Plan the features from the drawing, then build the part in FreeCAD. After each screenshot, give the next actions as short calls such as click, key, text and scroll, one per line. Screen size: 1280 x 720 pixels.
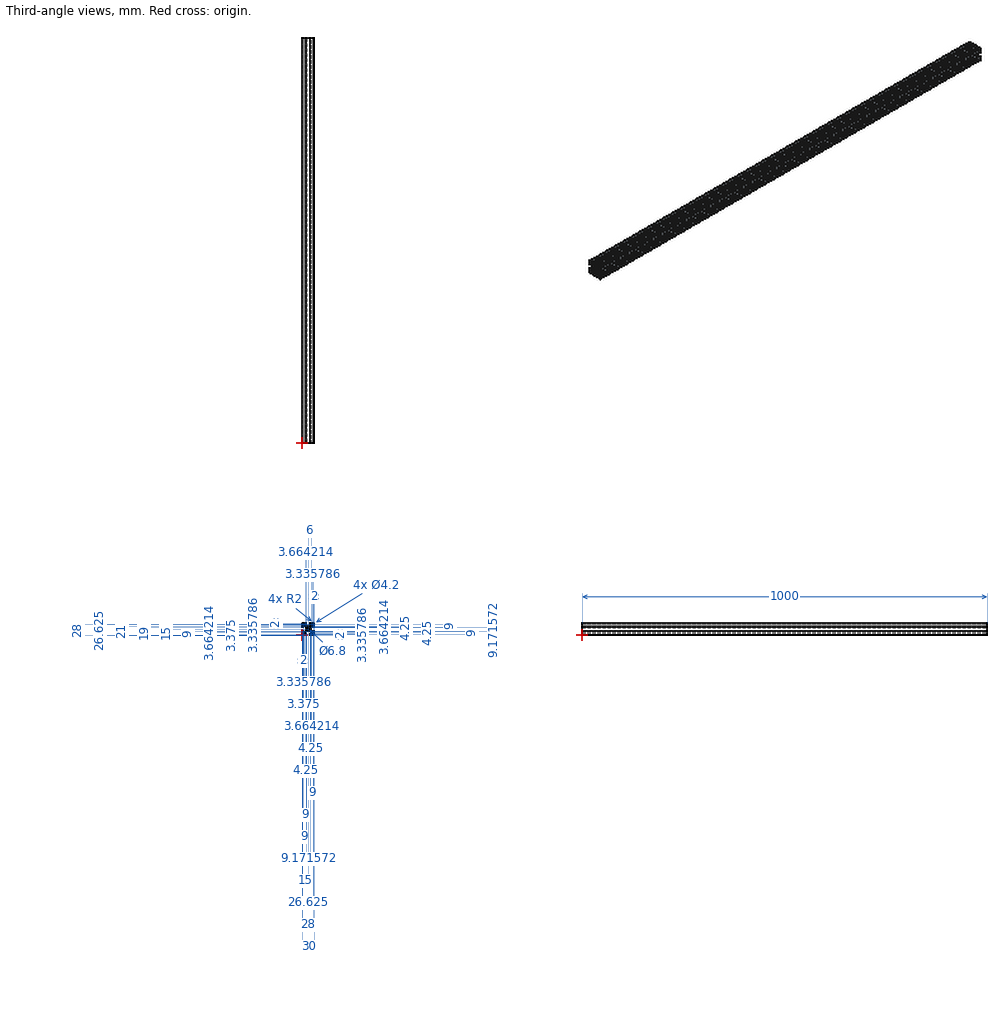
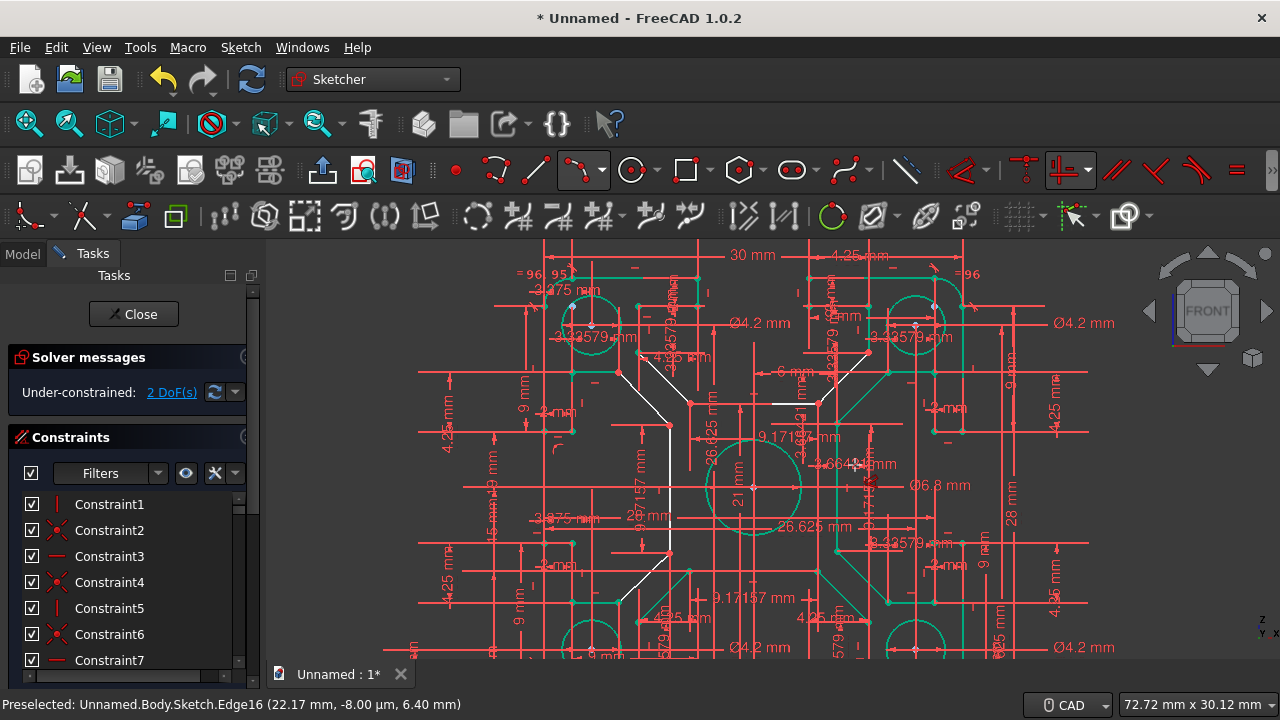
click(634, 588)
click(439, 595)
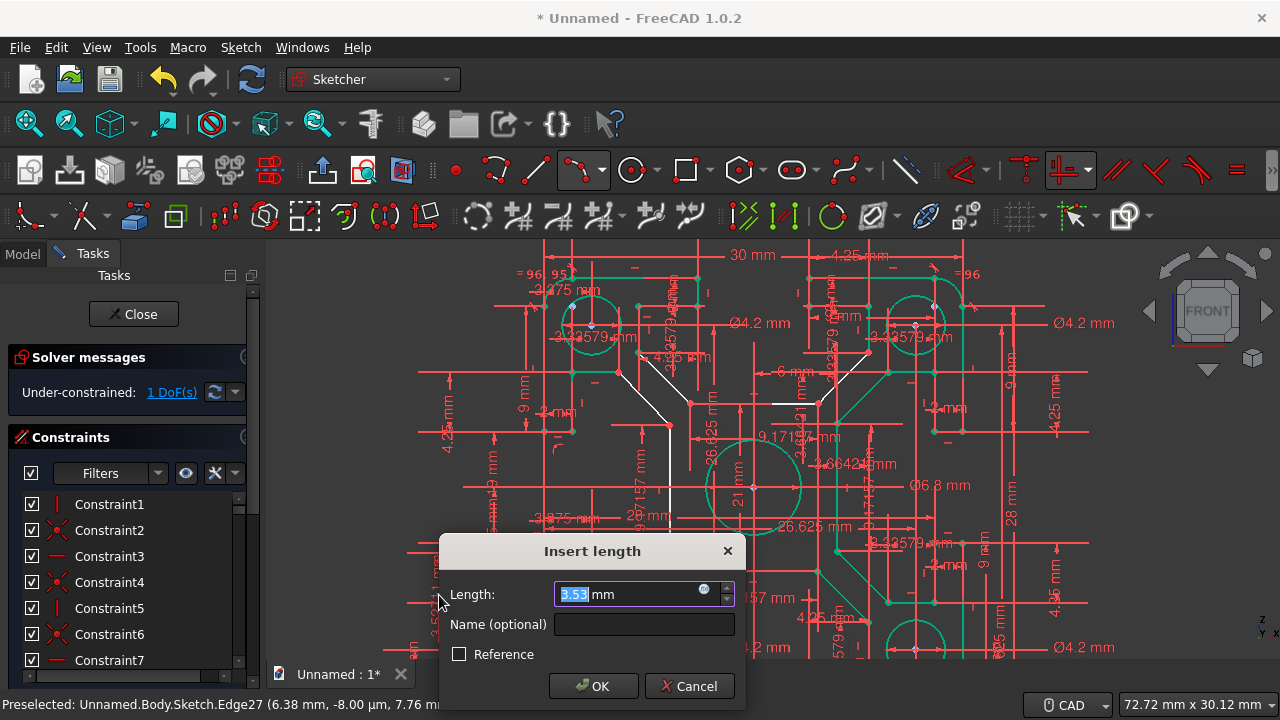
text(3.664214)
key(Return)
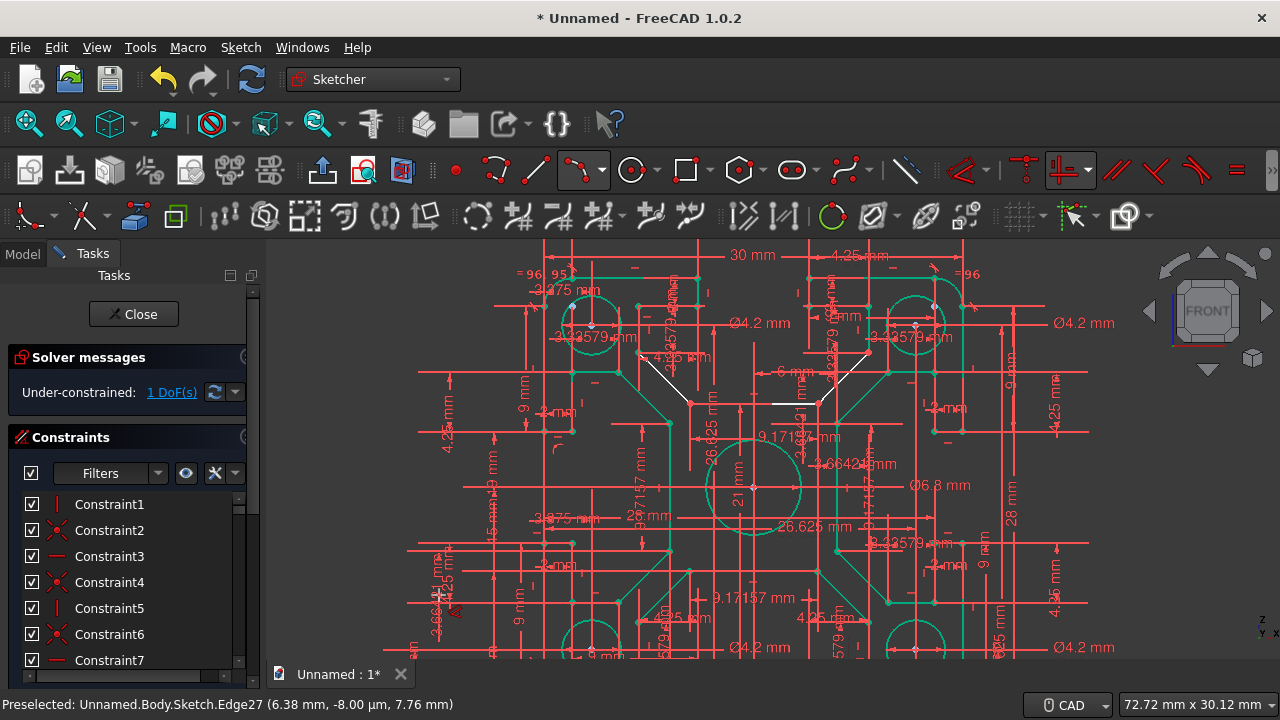
click(654, 368)
click(653, 462)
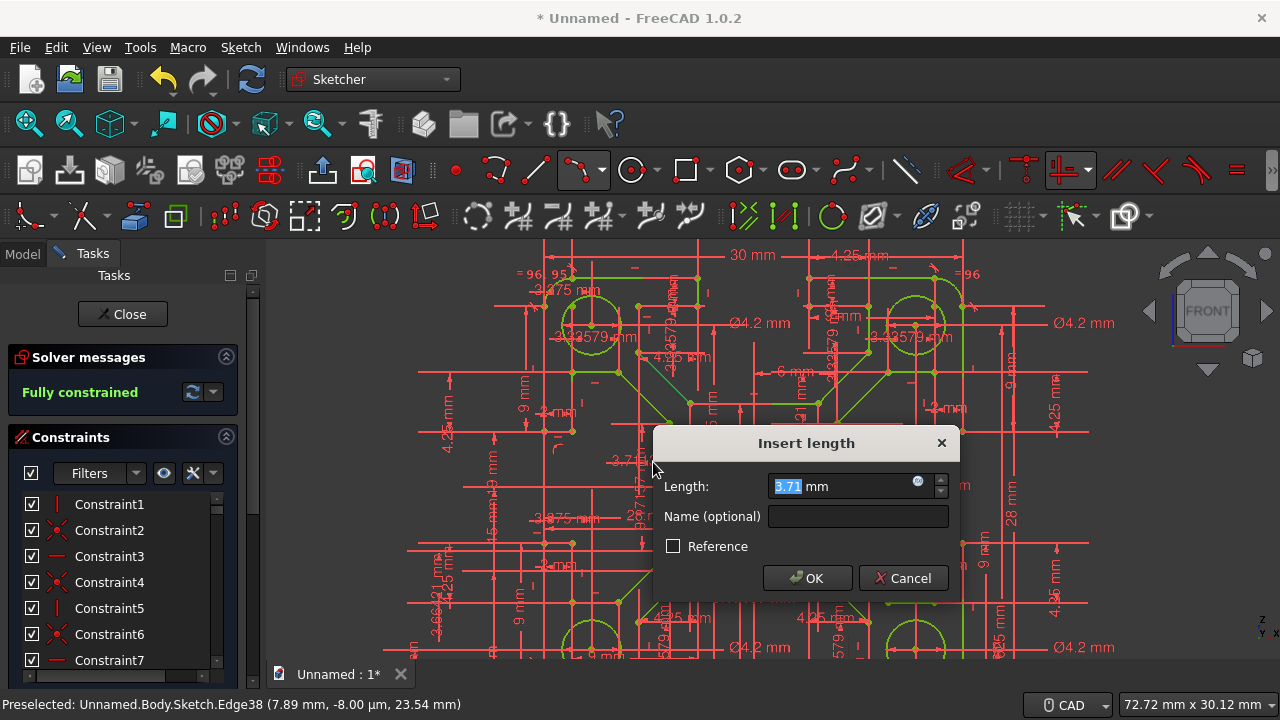
text(3.664214)
key(Return)
key(Escape)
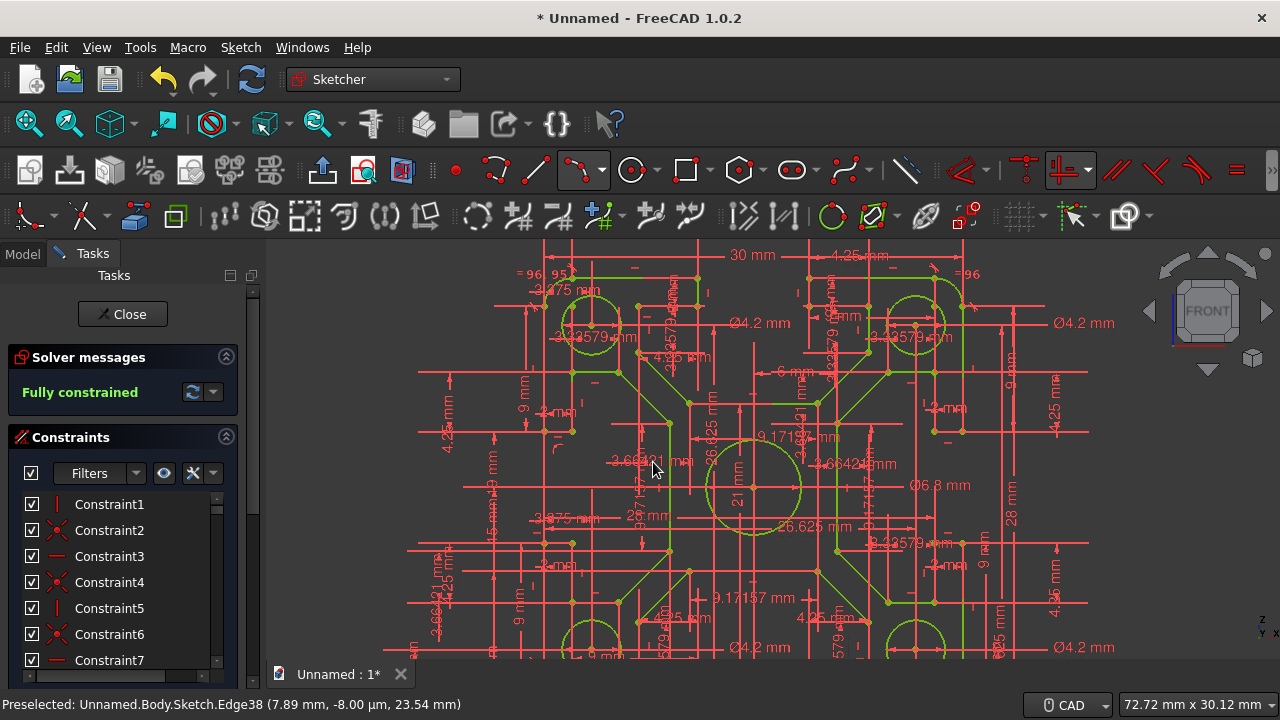
click(123, 314)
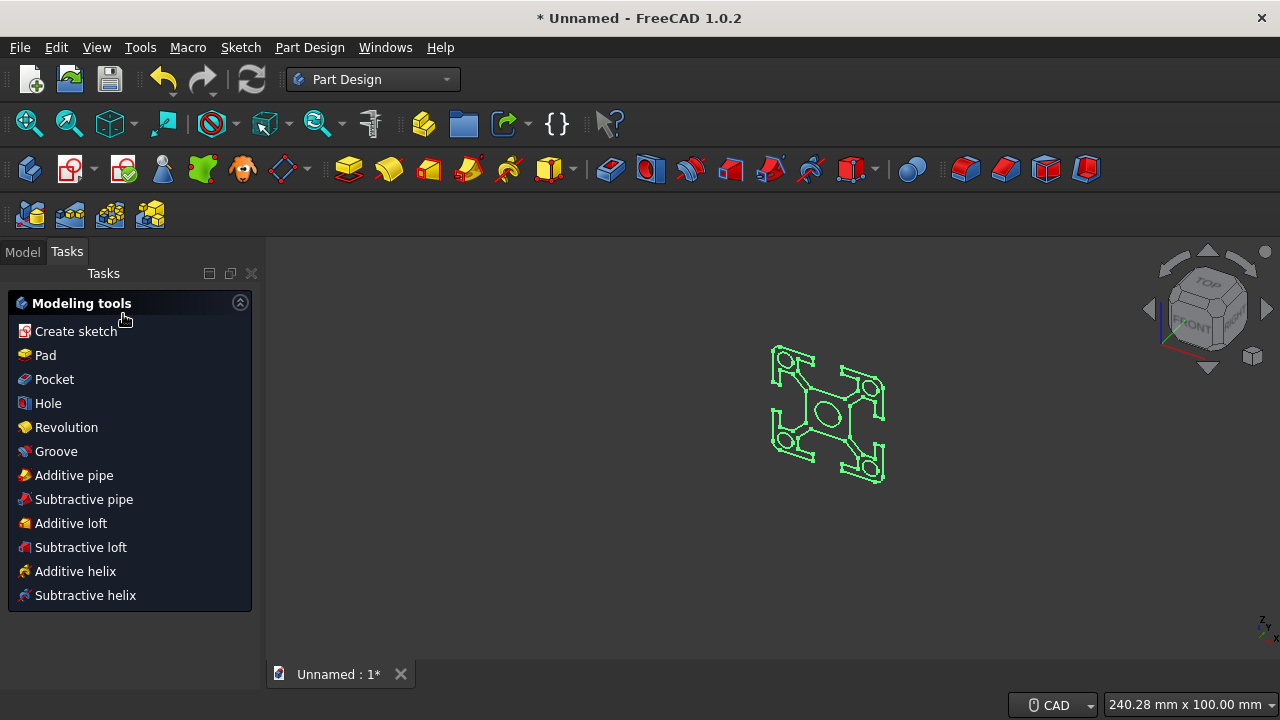
click(350, 170)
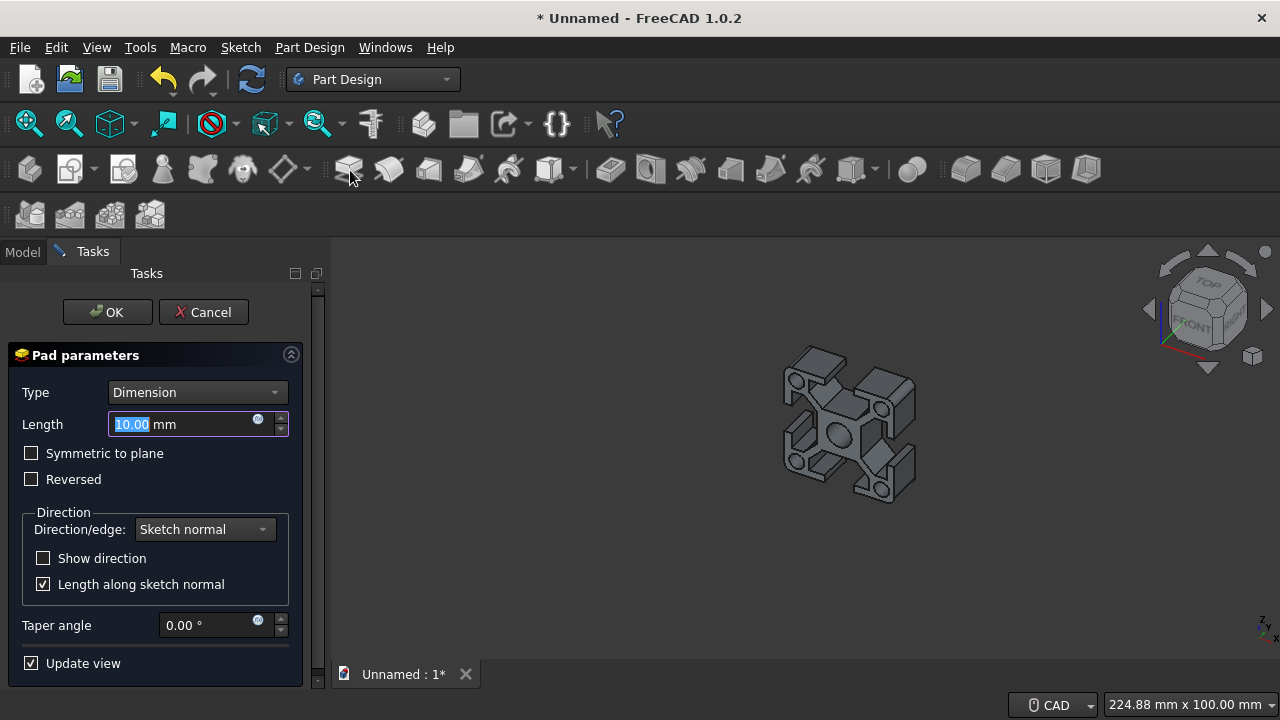
text(1000)
key(Tab)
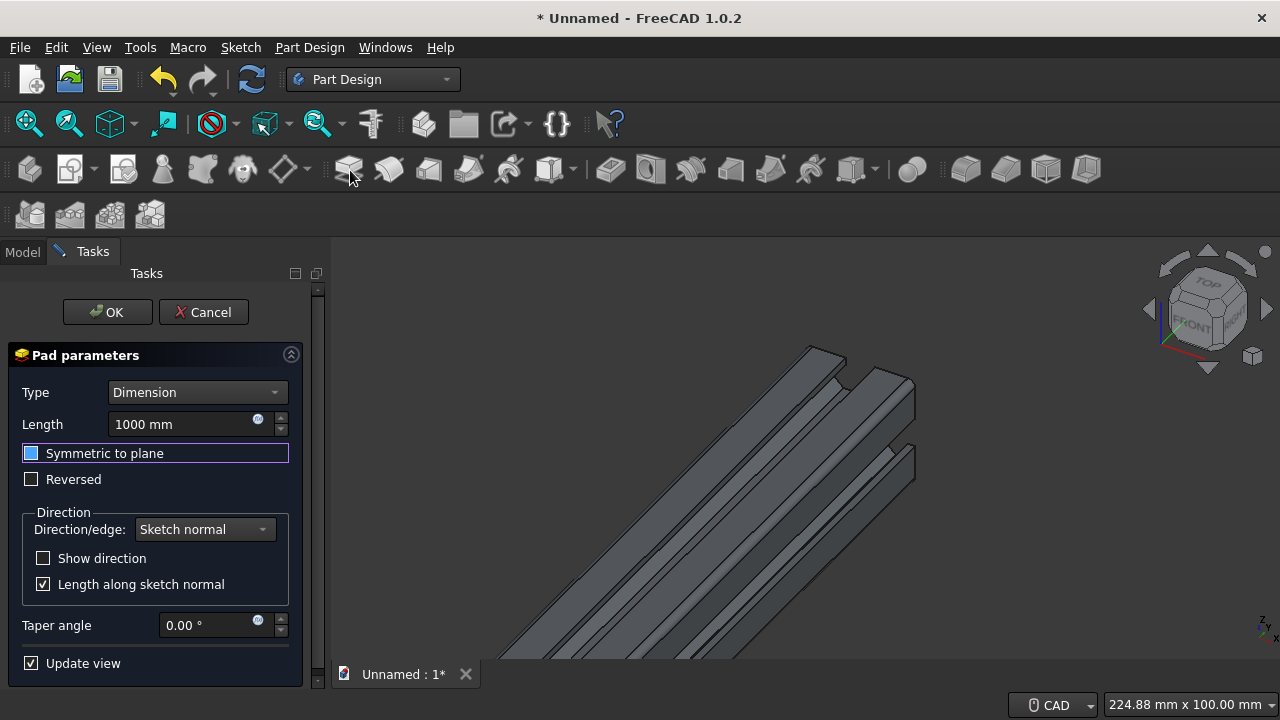
click(30, 479)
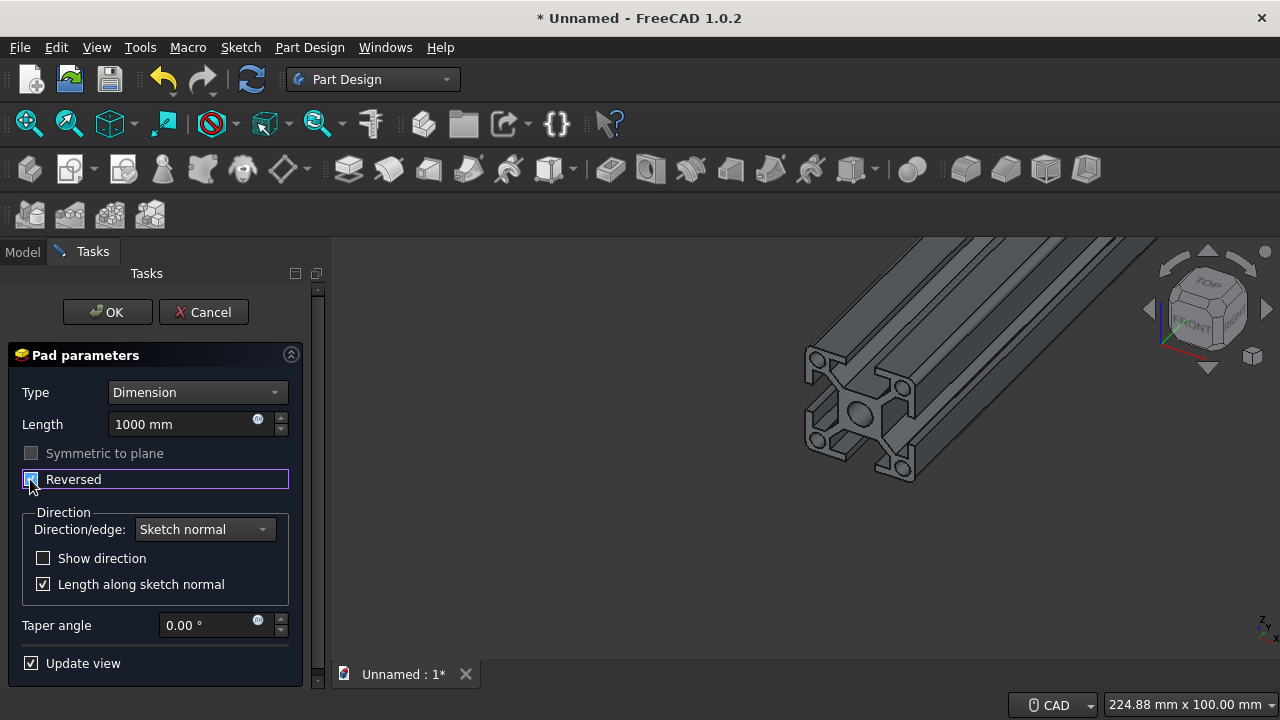
click(108, 312)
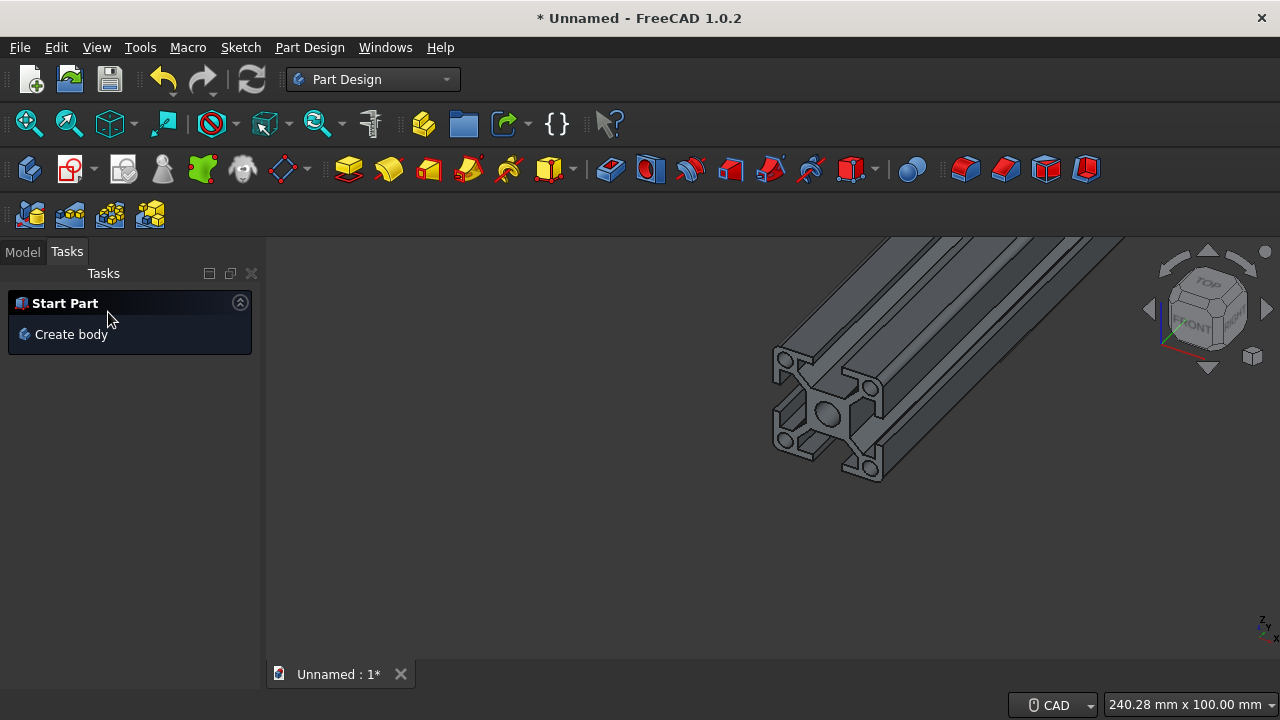
key(0)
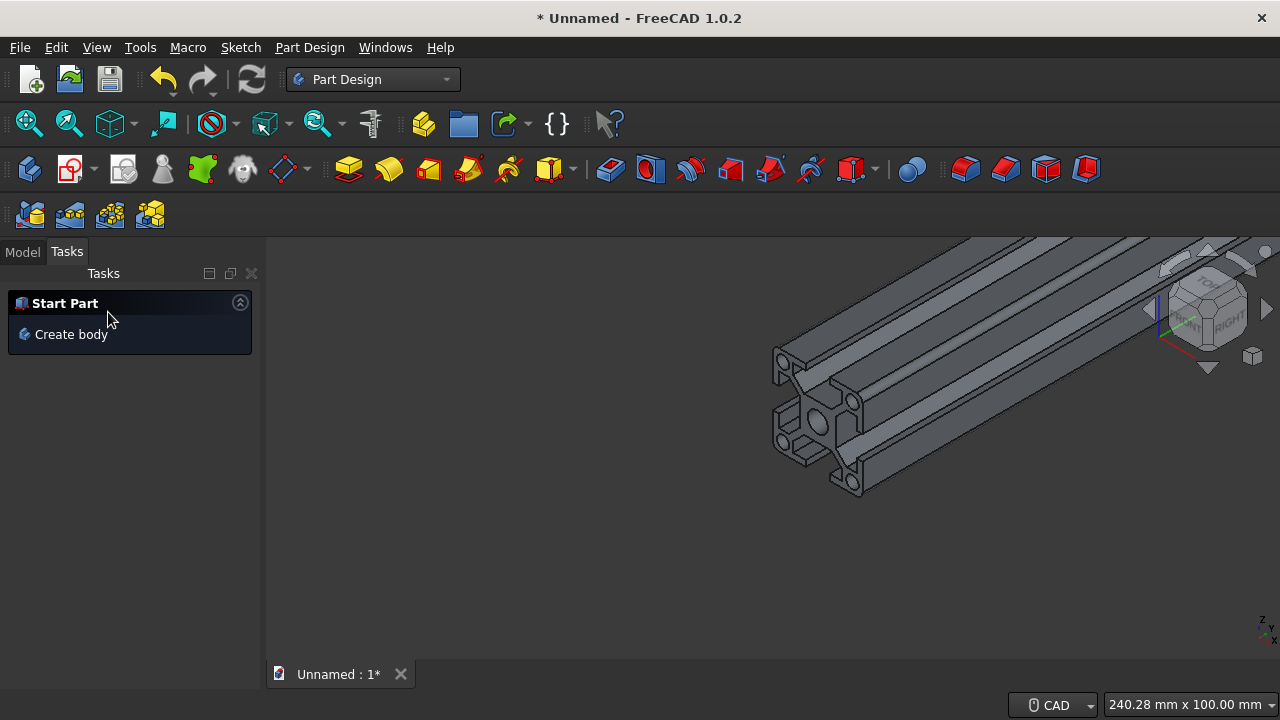
click(30, 124)